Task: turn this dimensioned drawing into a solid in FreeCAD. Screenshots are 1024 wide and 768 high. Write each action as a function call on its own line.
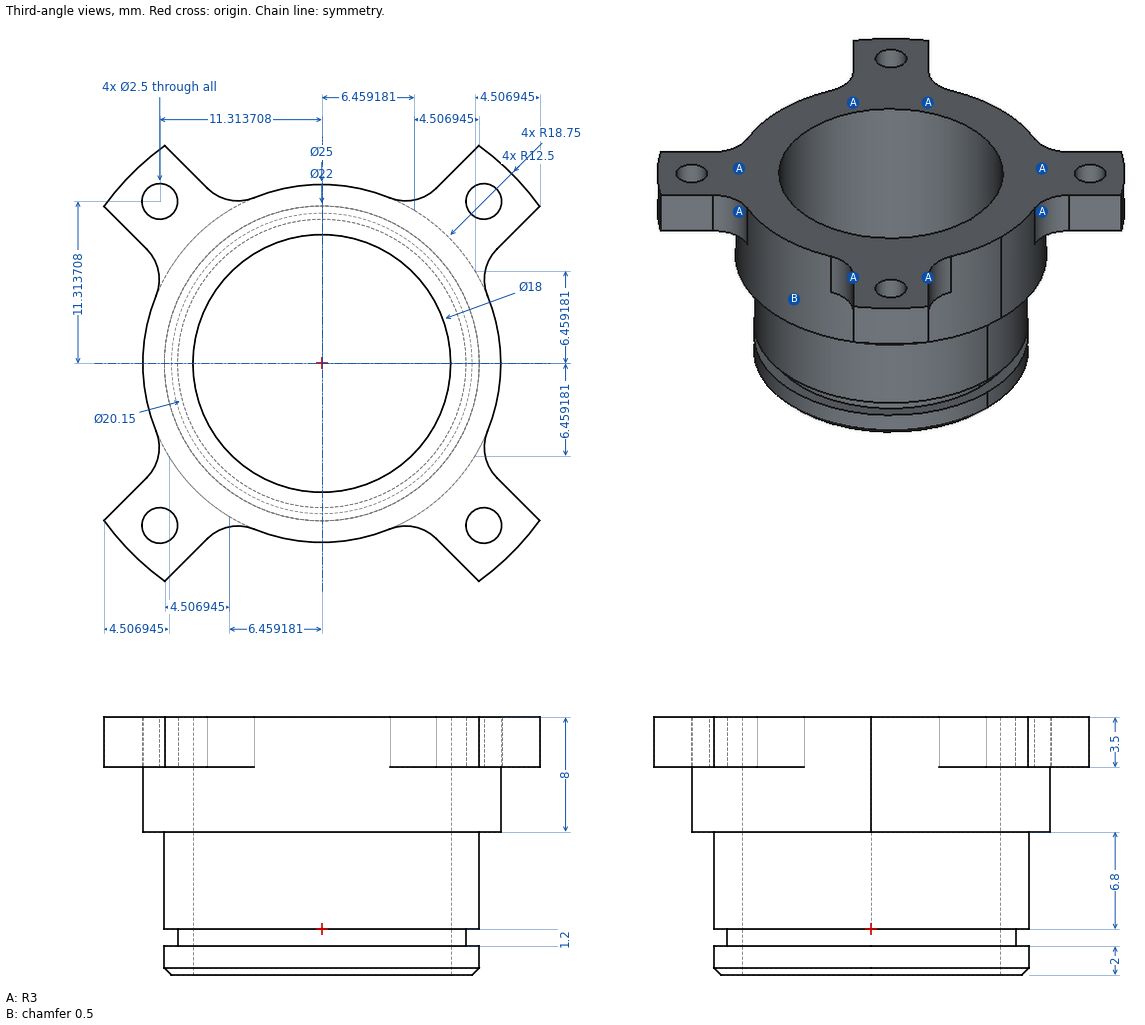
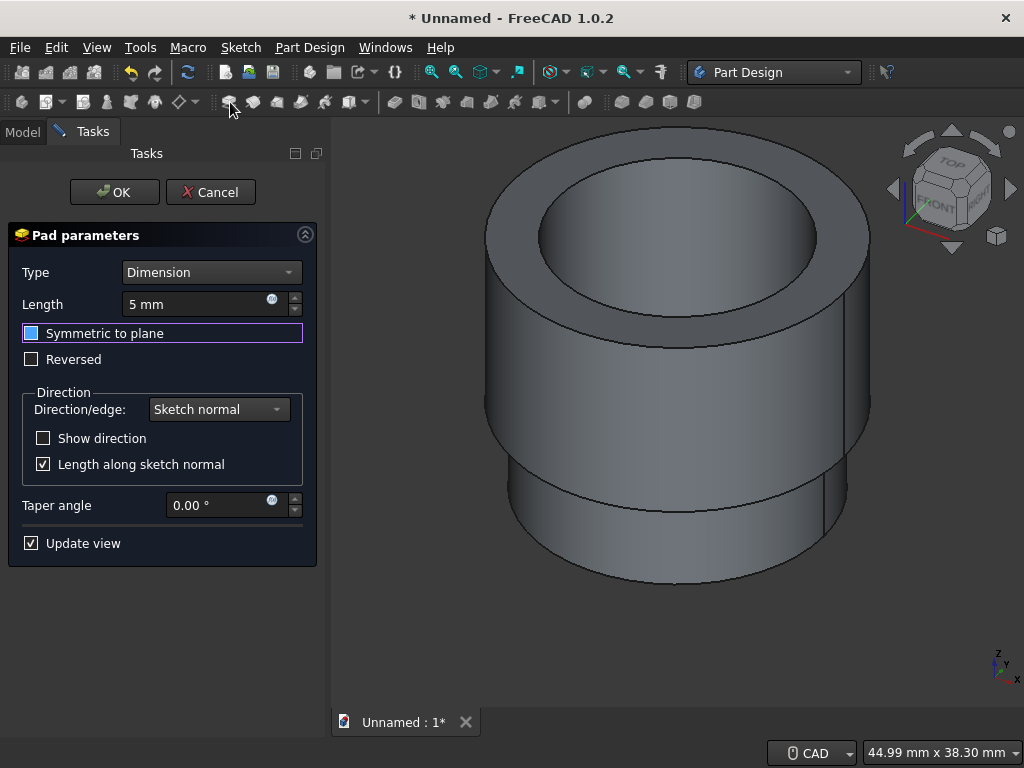
click(115, 192)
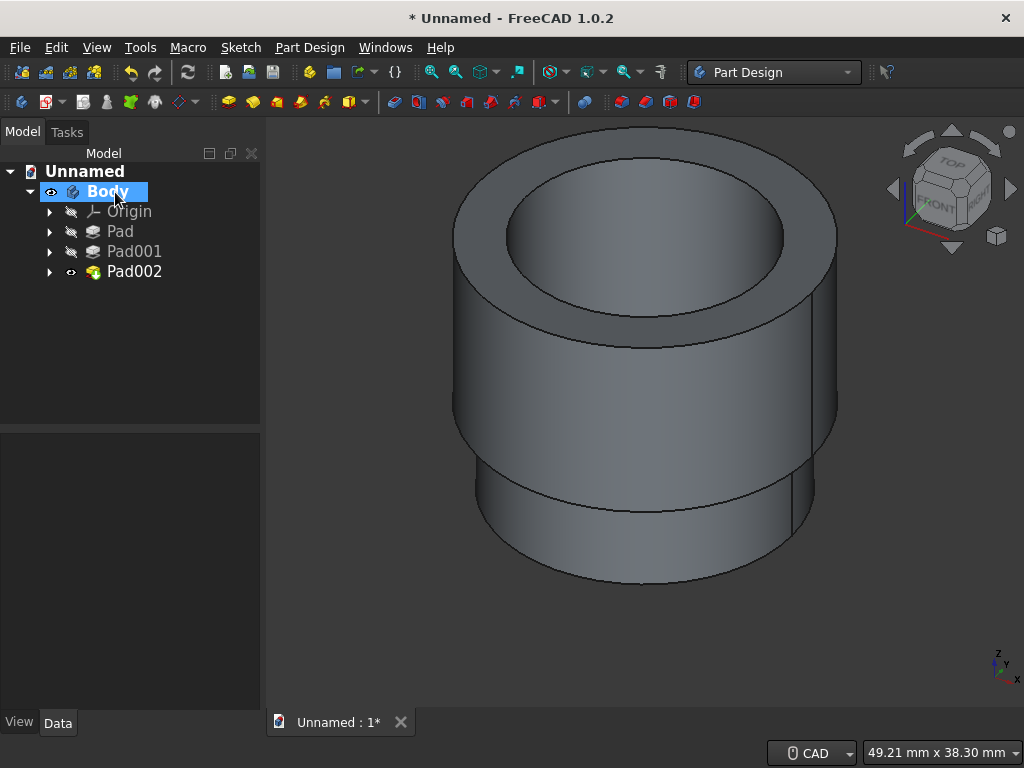
click(432, 72)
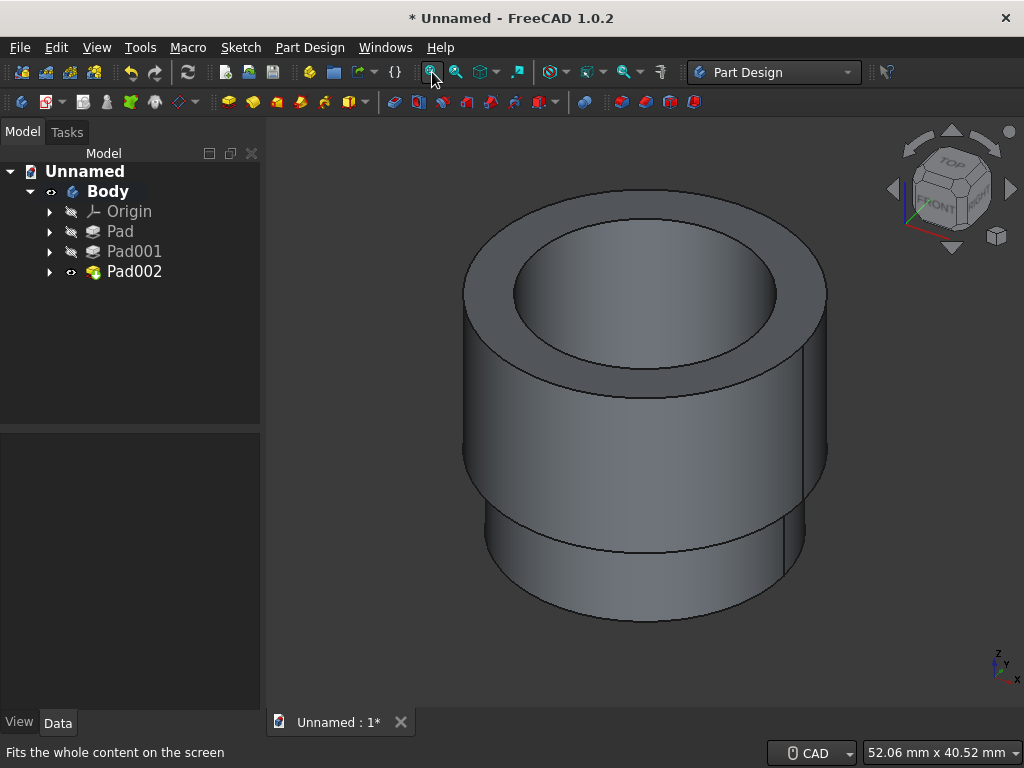
click(50, 212)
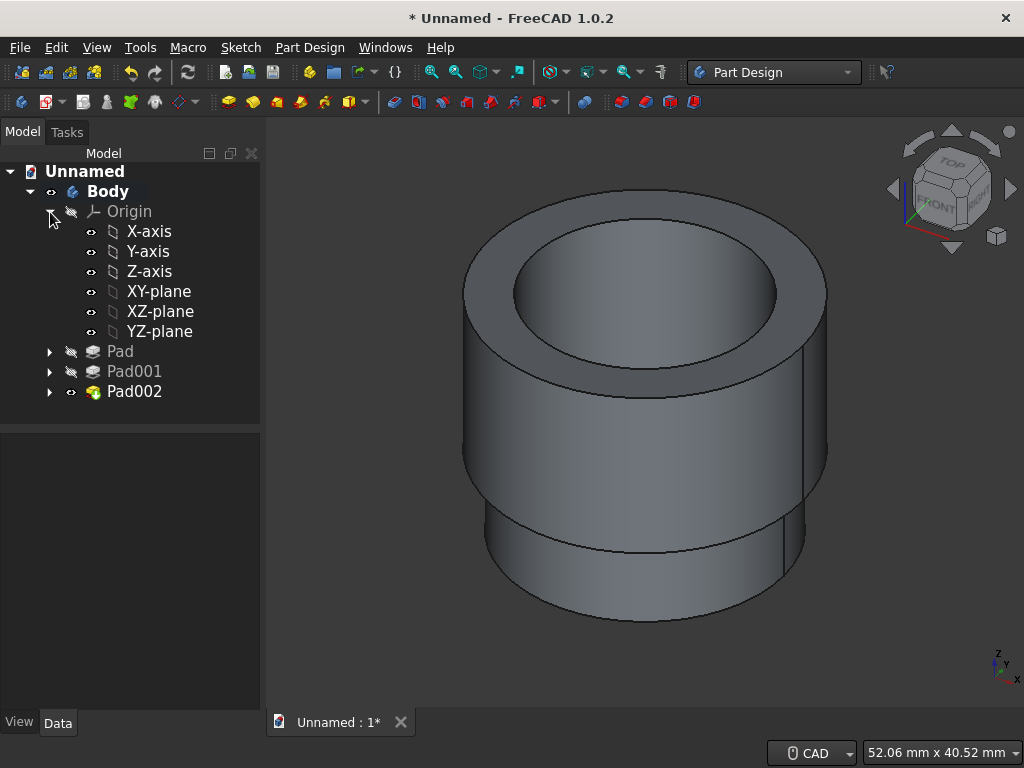
click(136, 292)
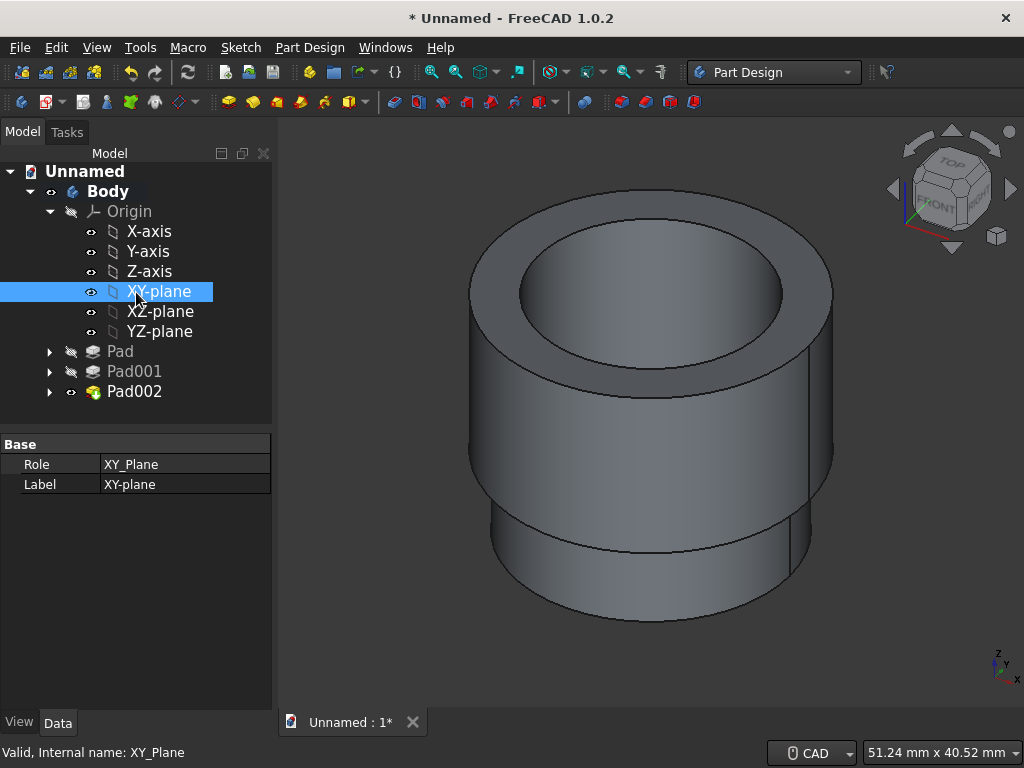
click(180, 102)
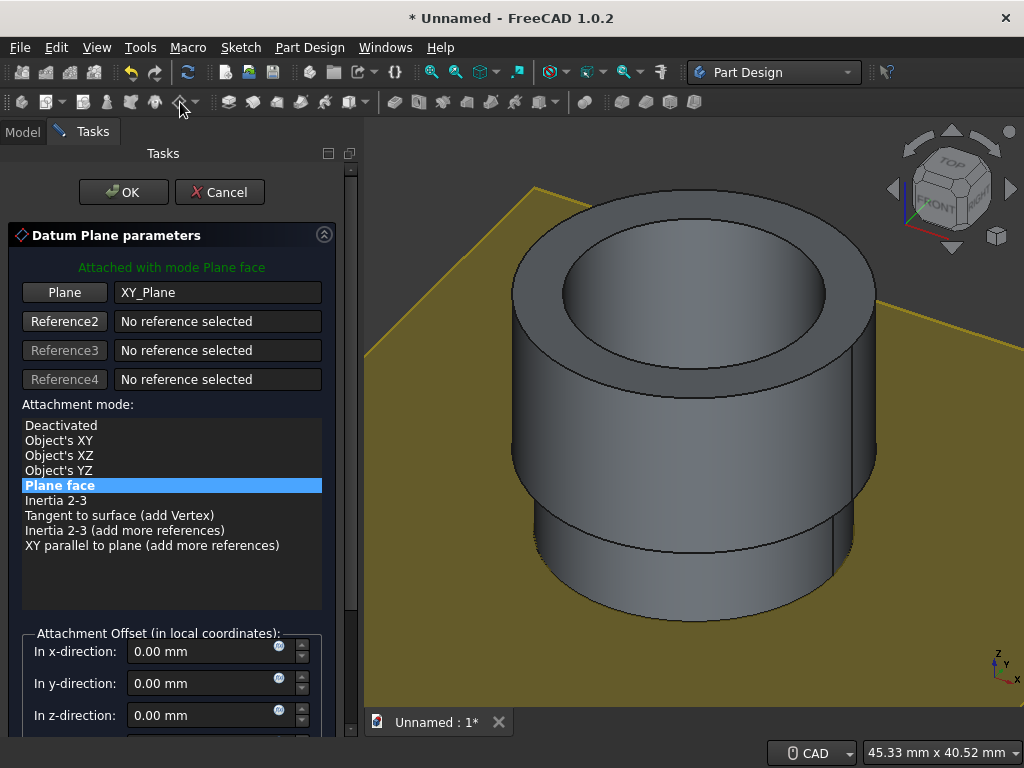
triple_click(210, 715)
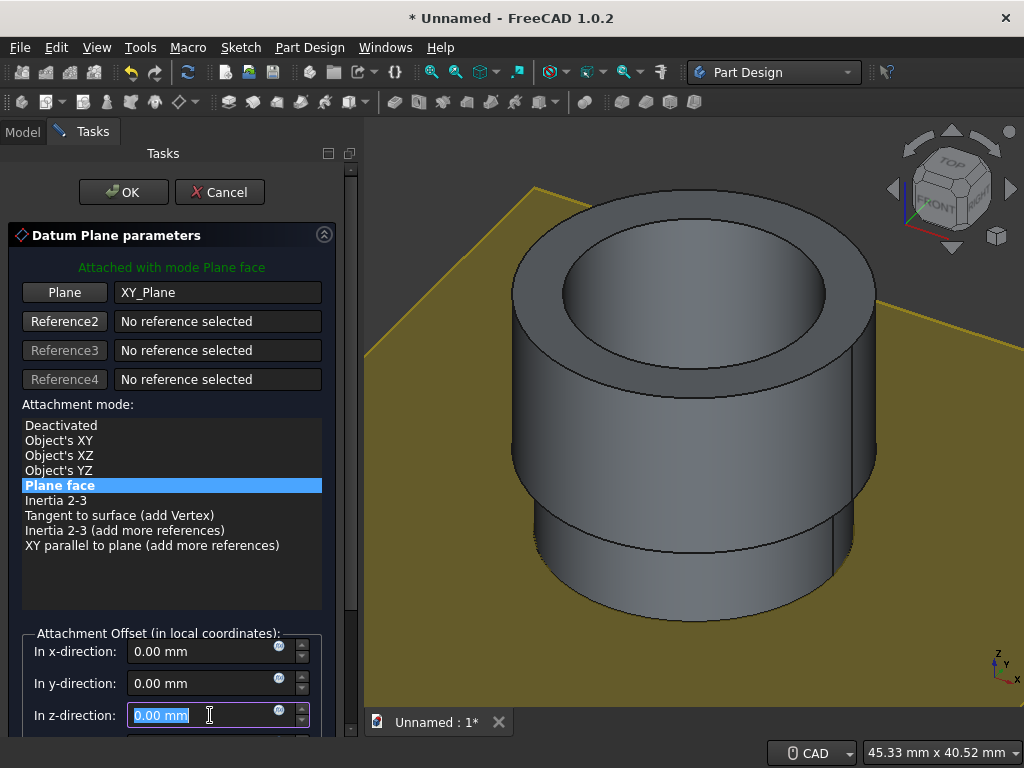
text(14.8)
key(Tab)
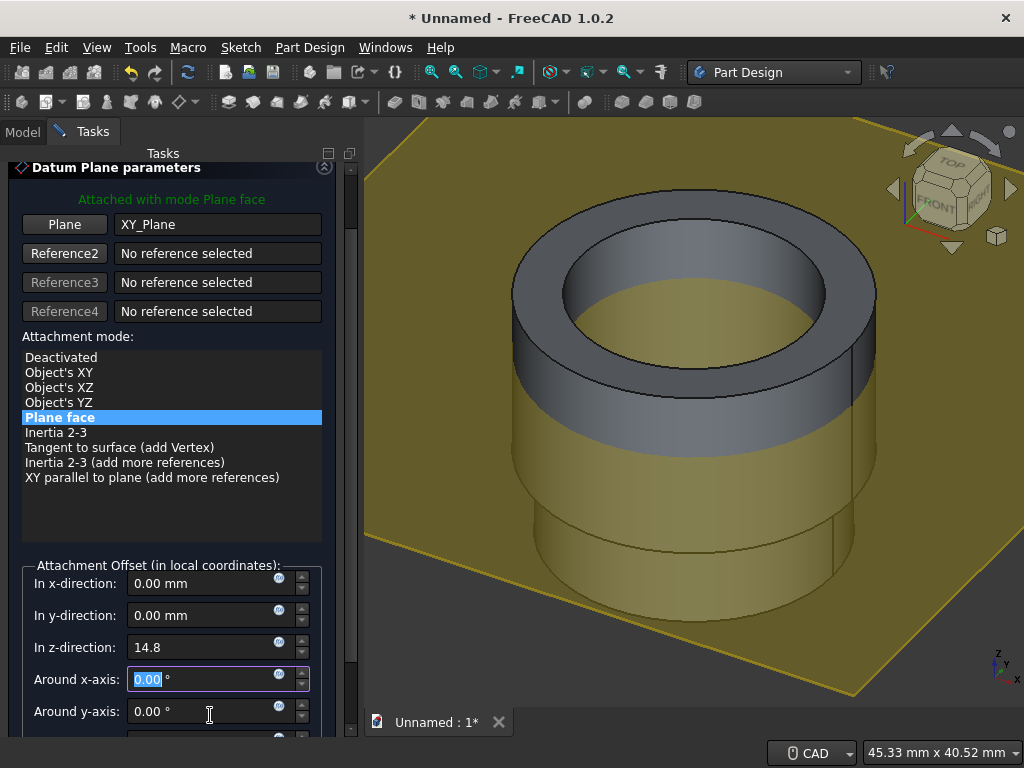
scroll(351, 450, up, 2)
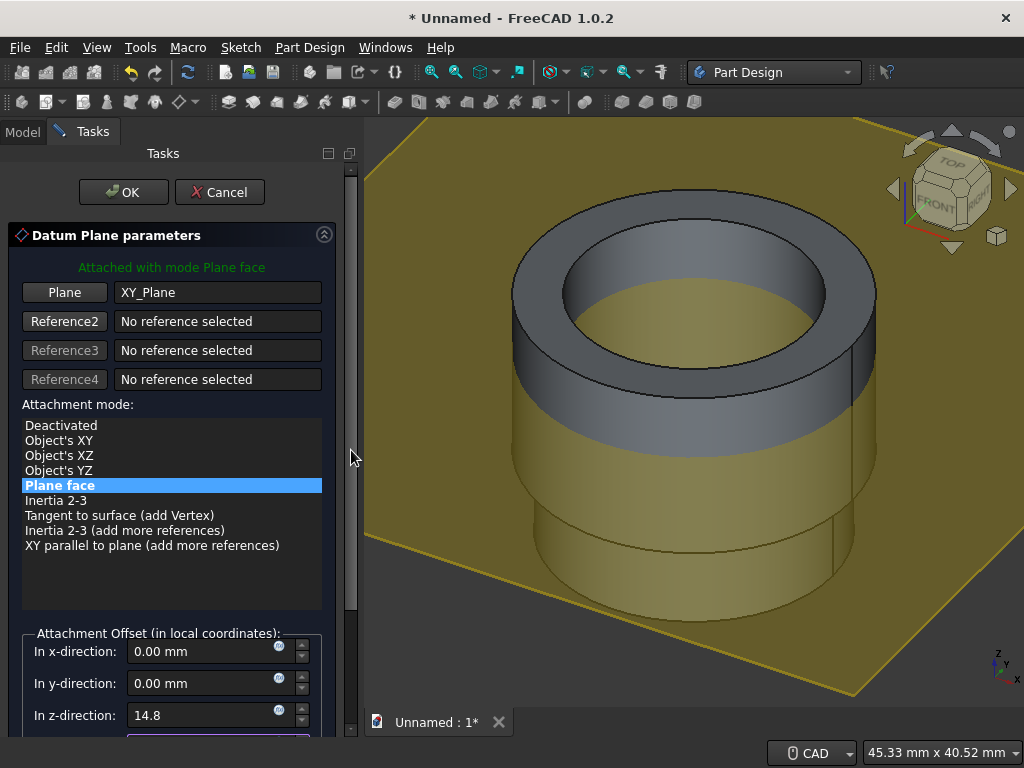
click(124, 192)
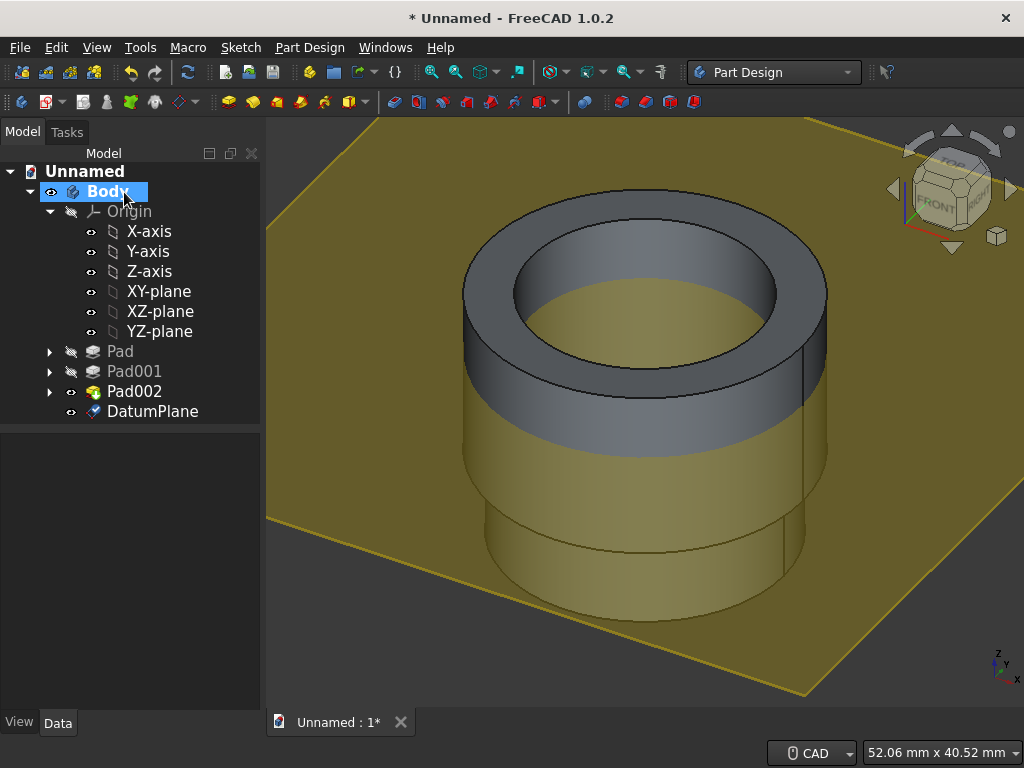
click(116, 412)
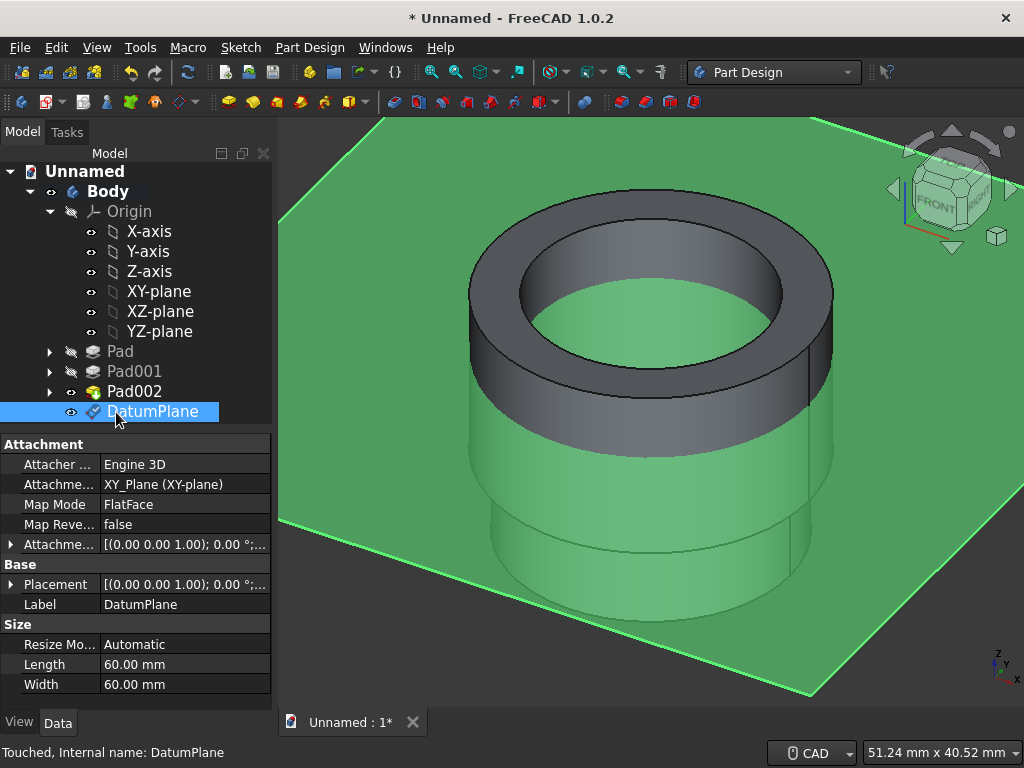
click(46, 102)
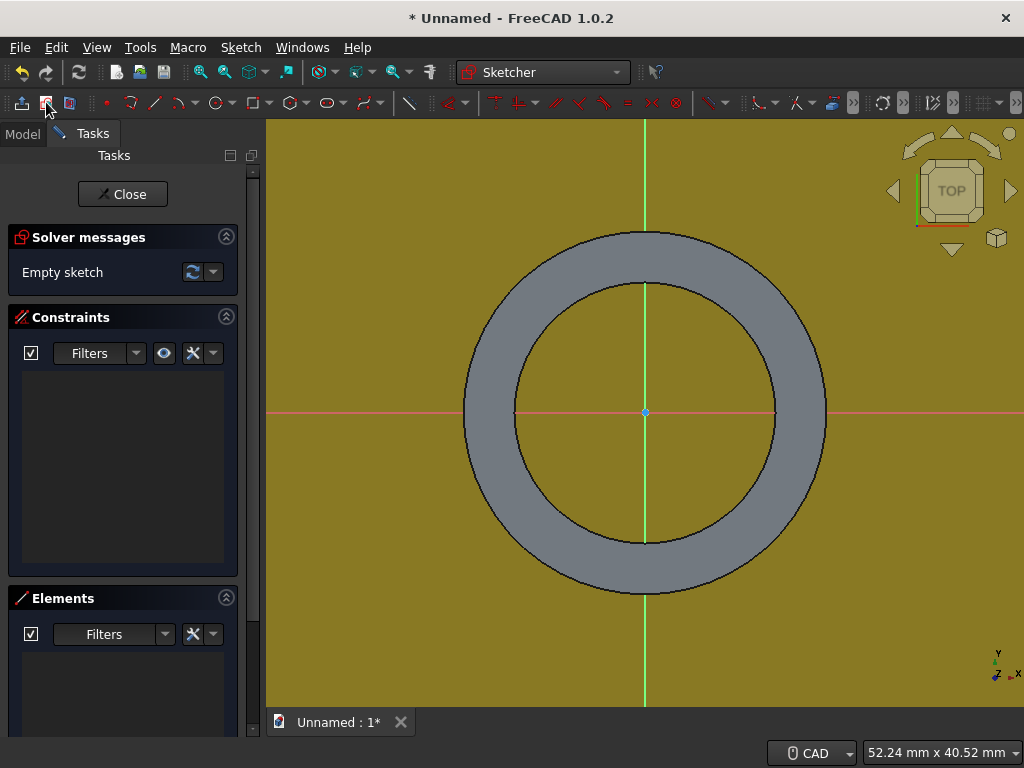
click(70, 104)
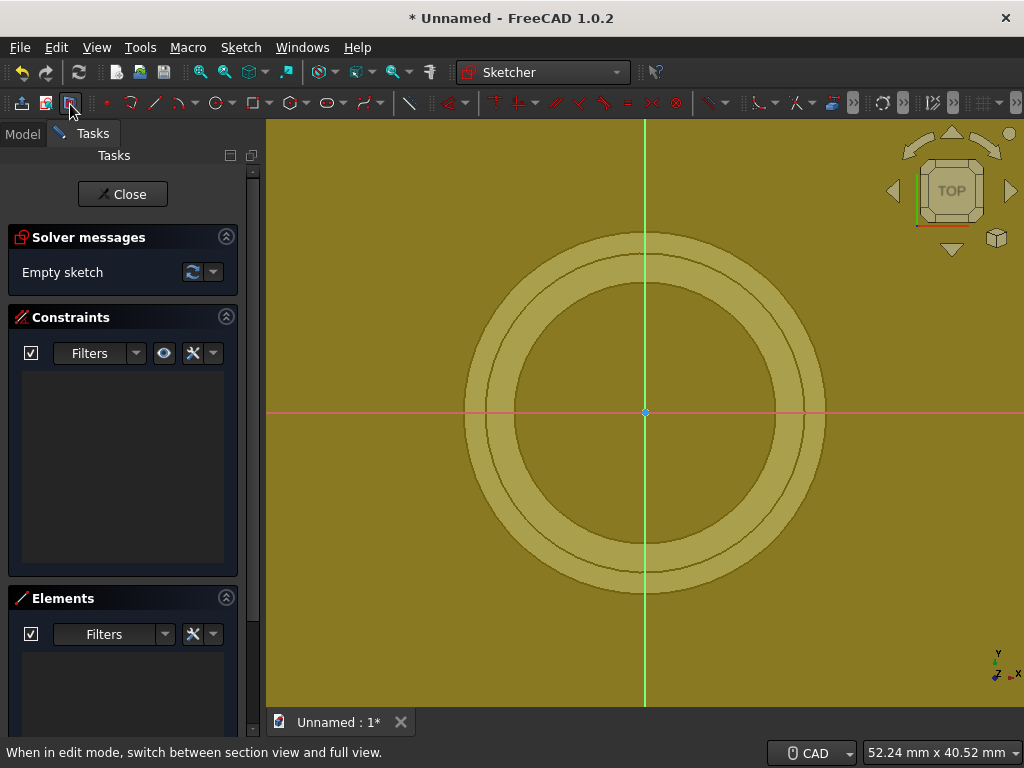
click(216, 104)